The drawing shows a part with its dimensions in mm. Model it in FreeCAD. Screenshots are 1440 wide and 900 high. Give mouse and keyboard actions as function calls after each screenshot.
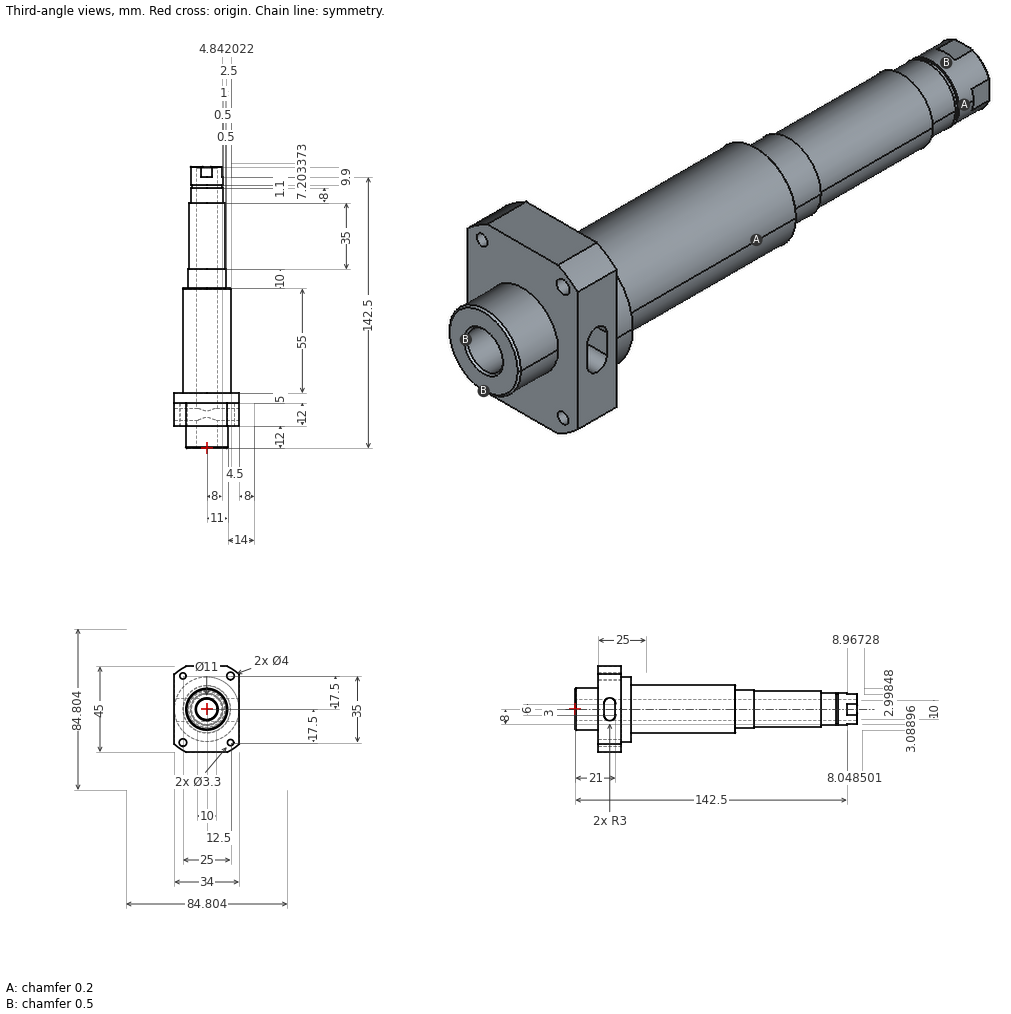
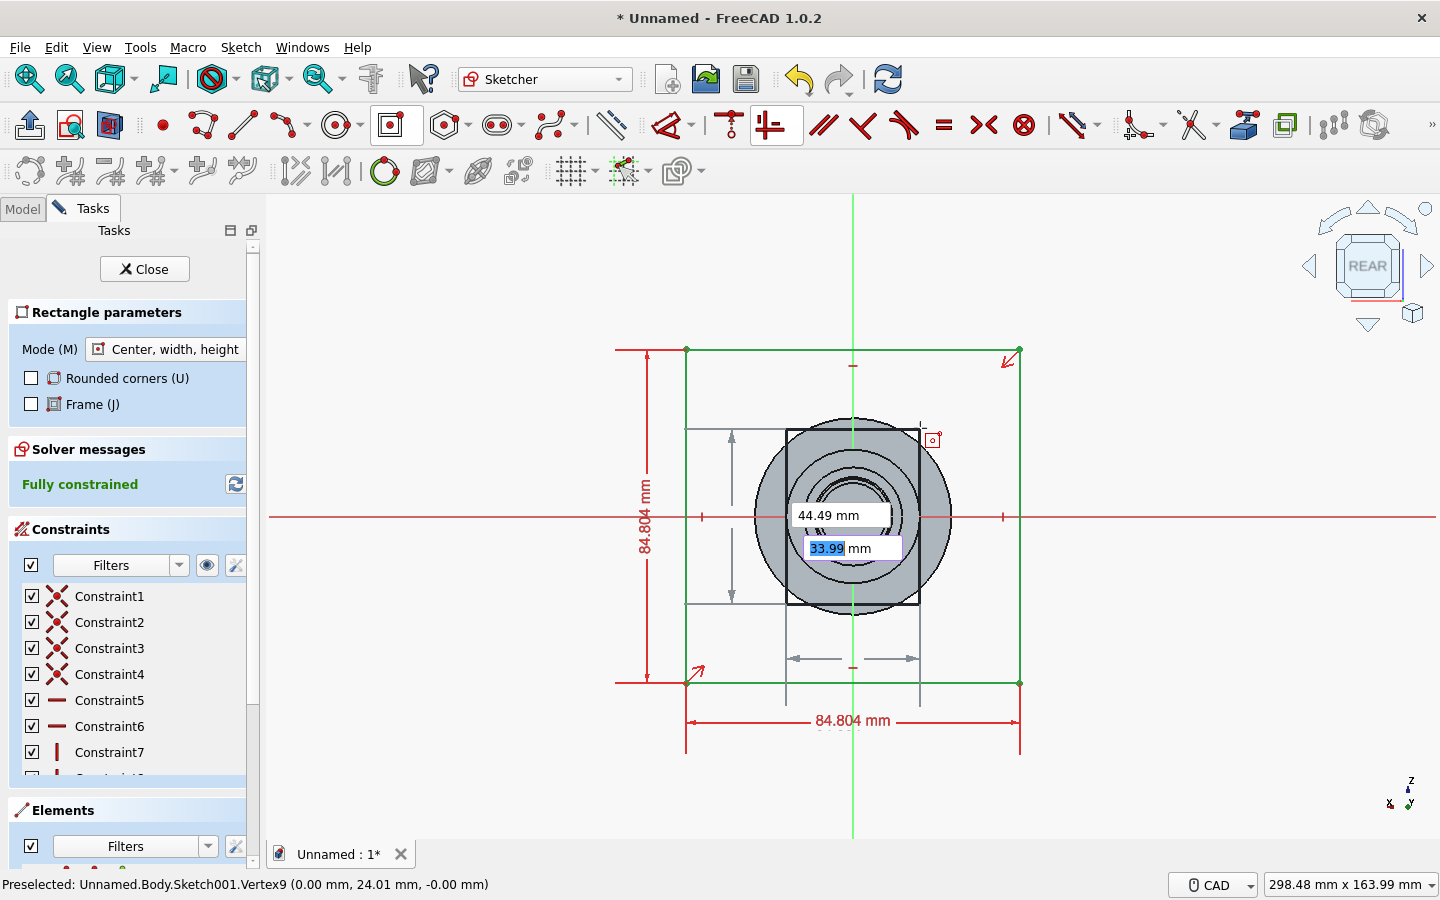
text(34)
key(Tab)
text(45)
key(Return)
key(Escape)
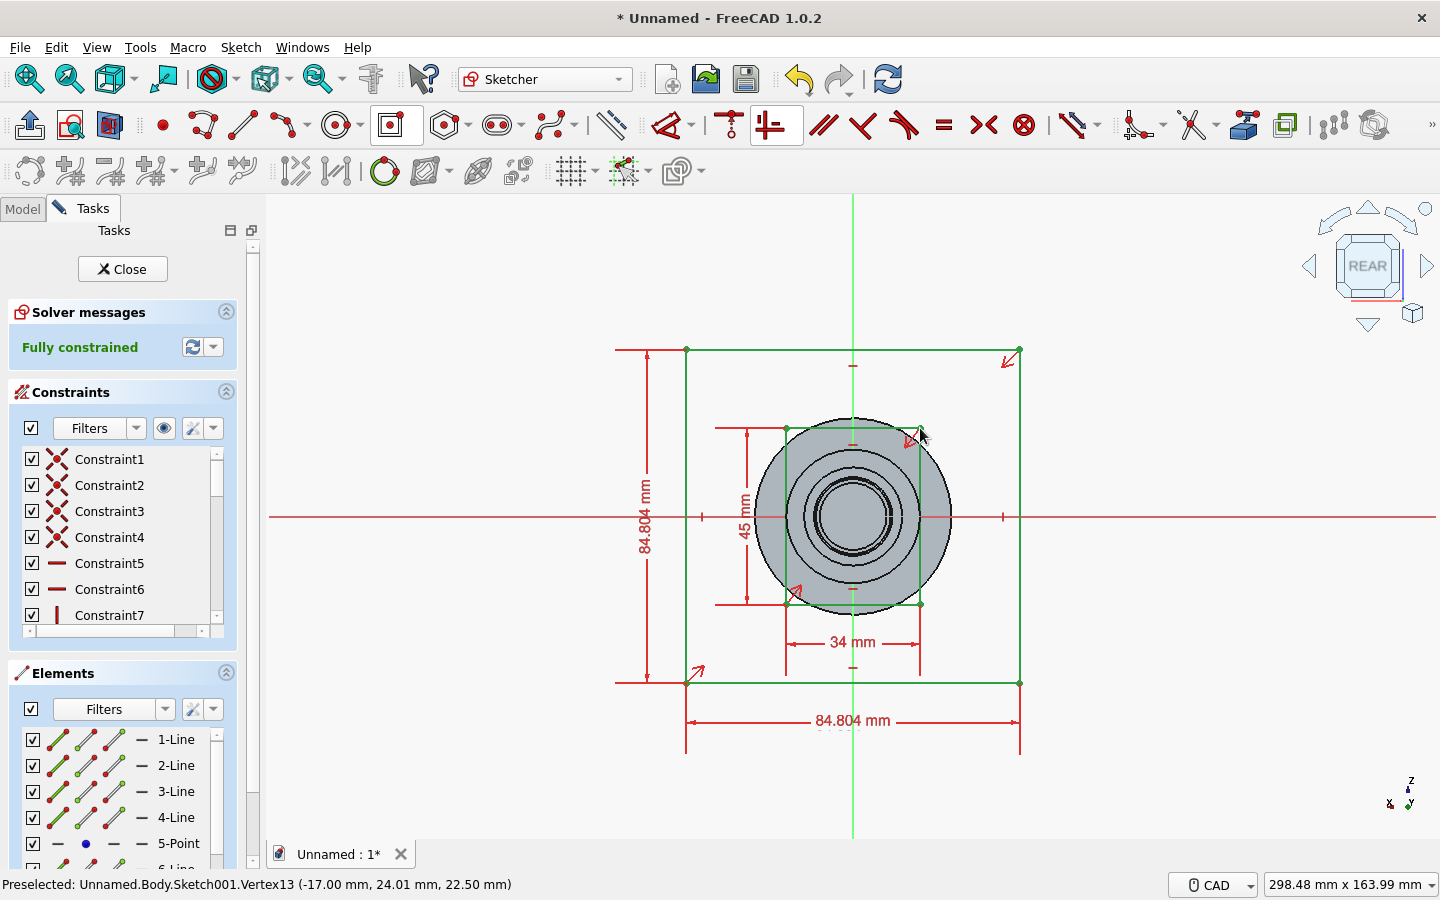
click(123, 269)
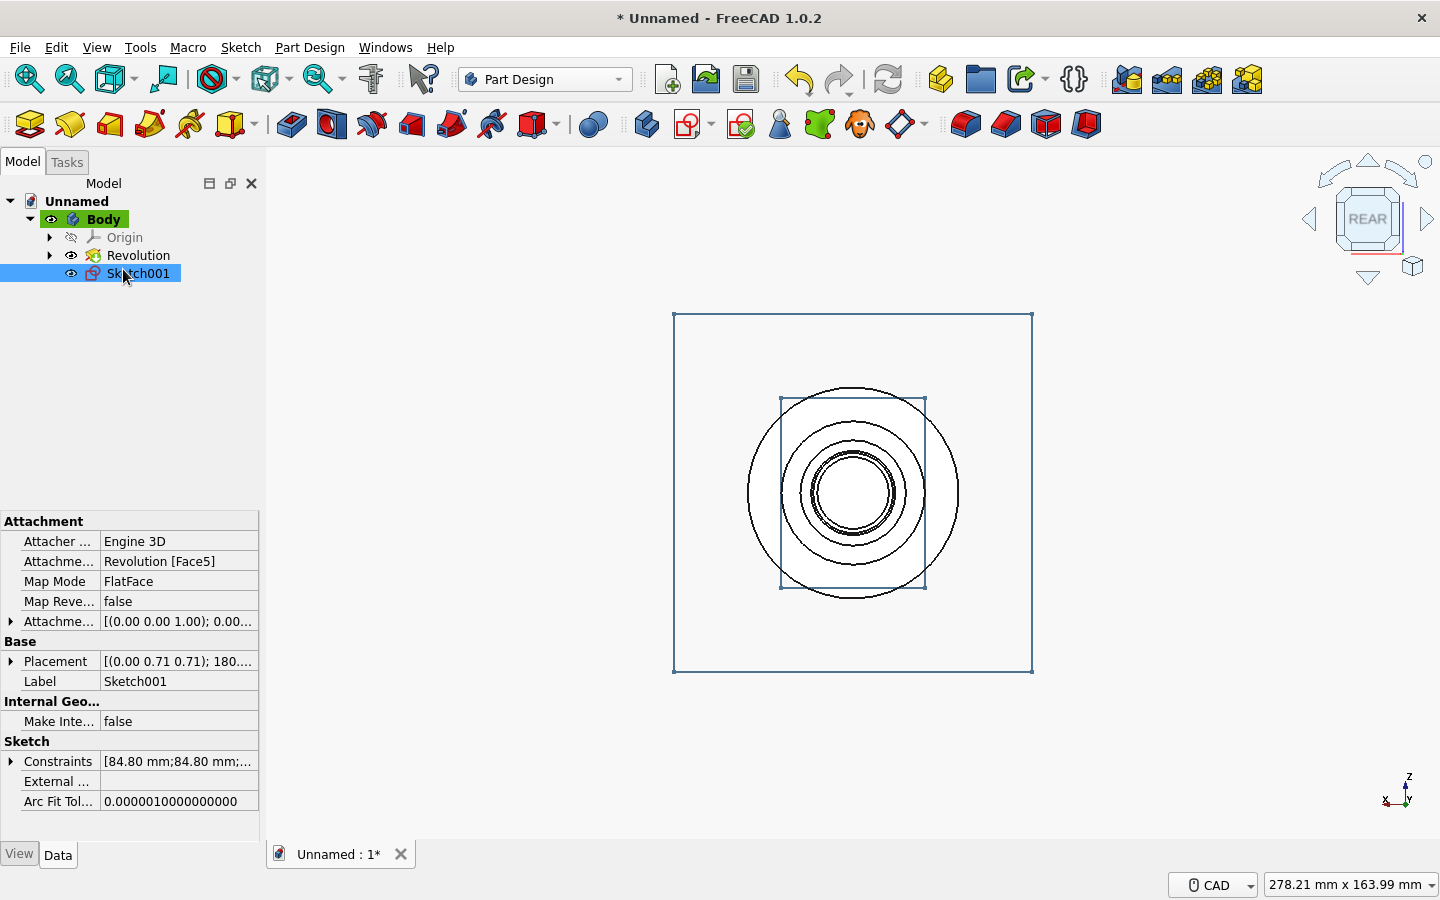
click(292, 124)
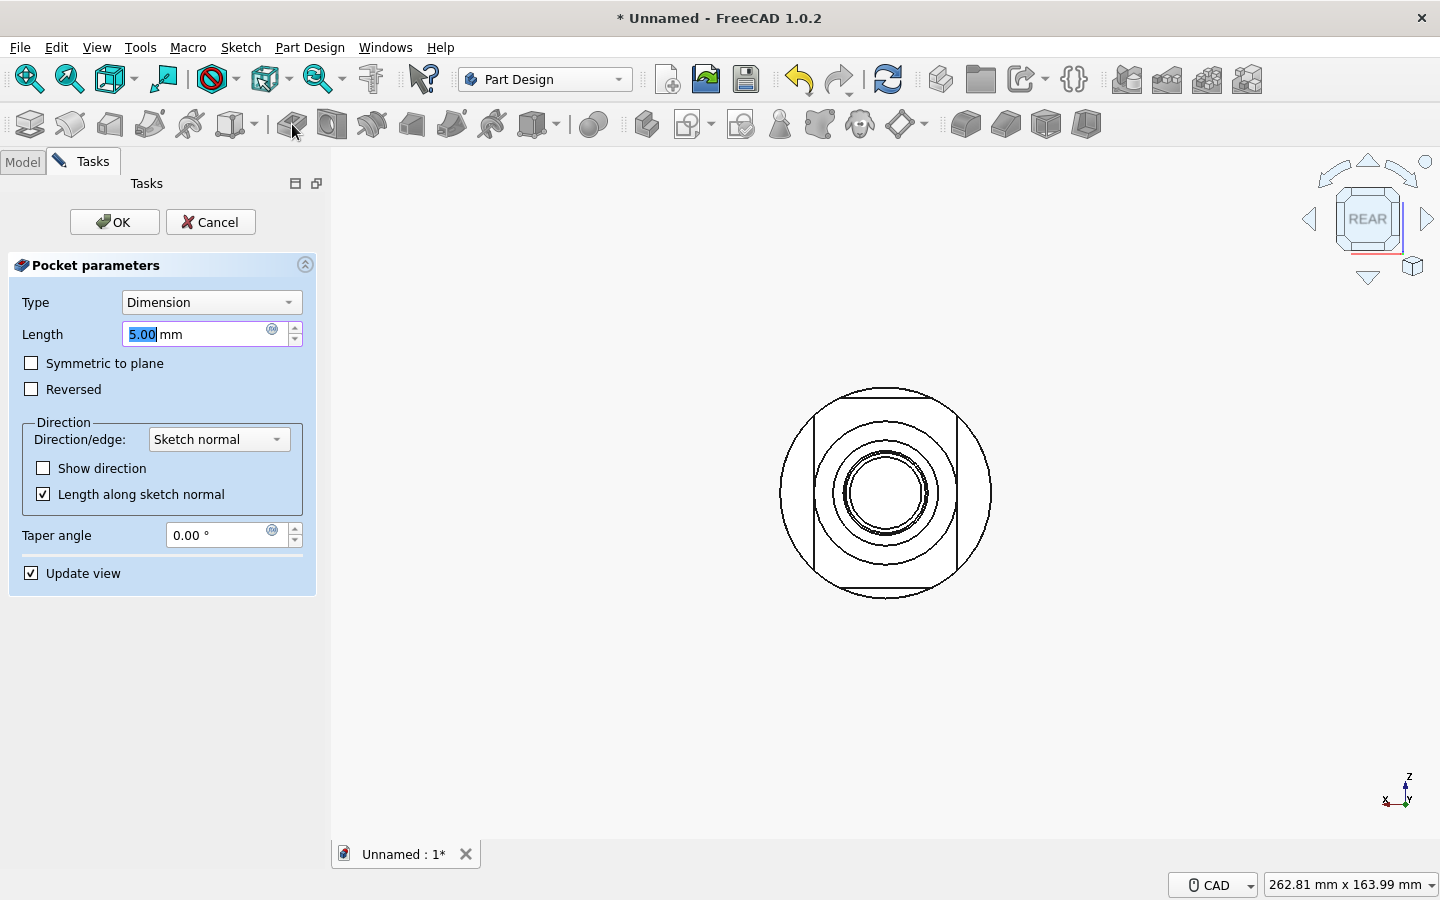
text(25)
key(Tab)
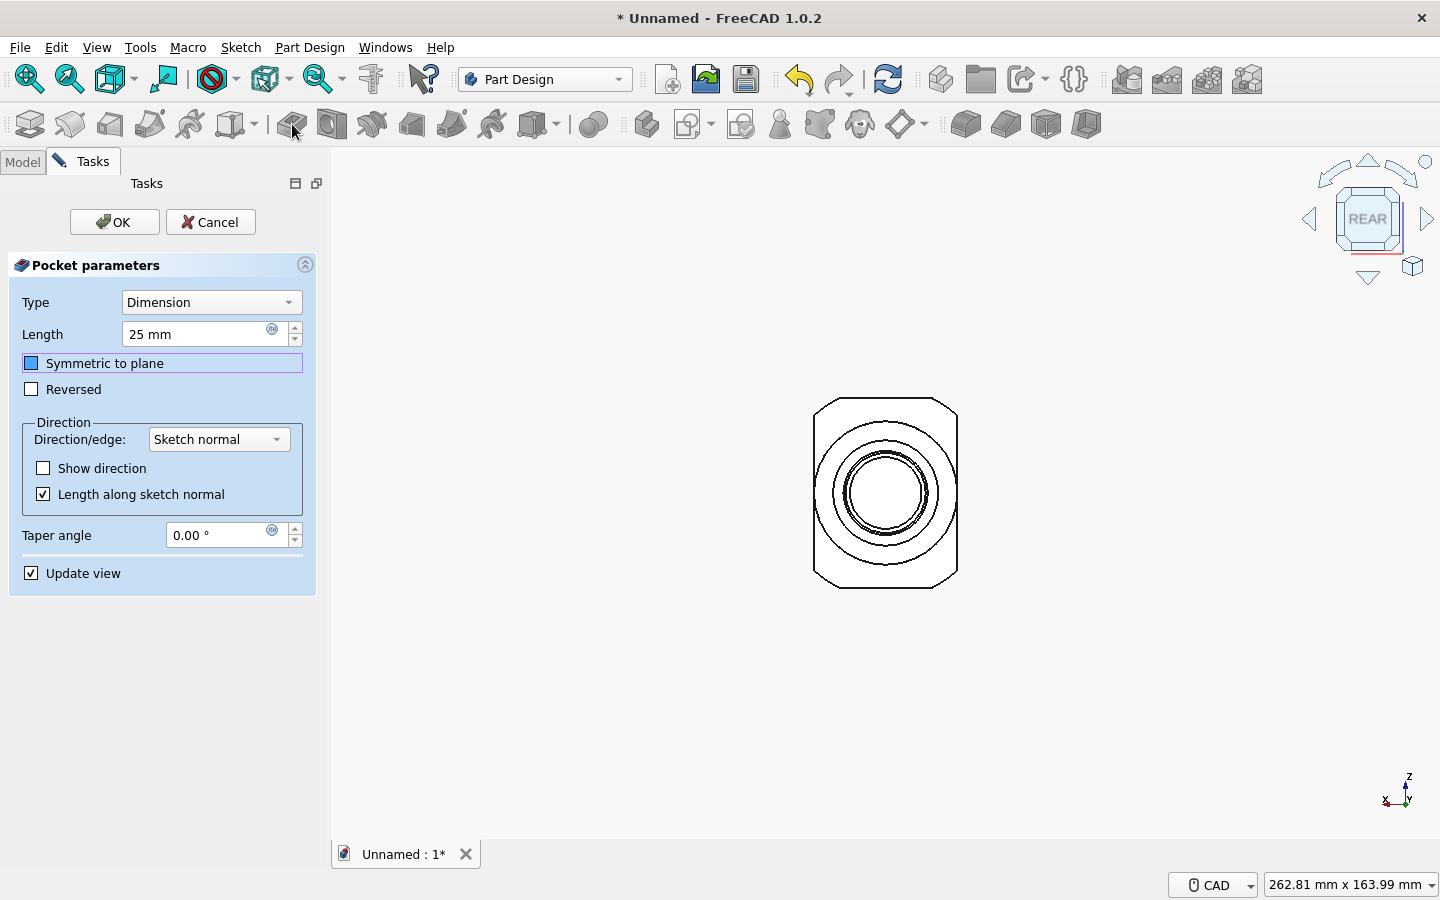
click(115, 222)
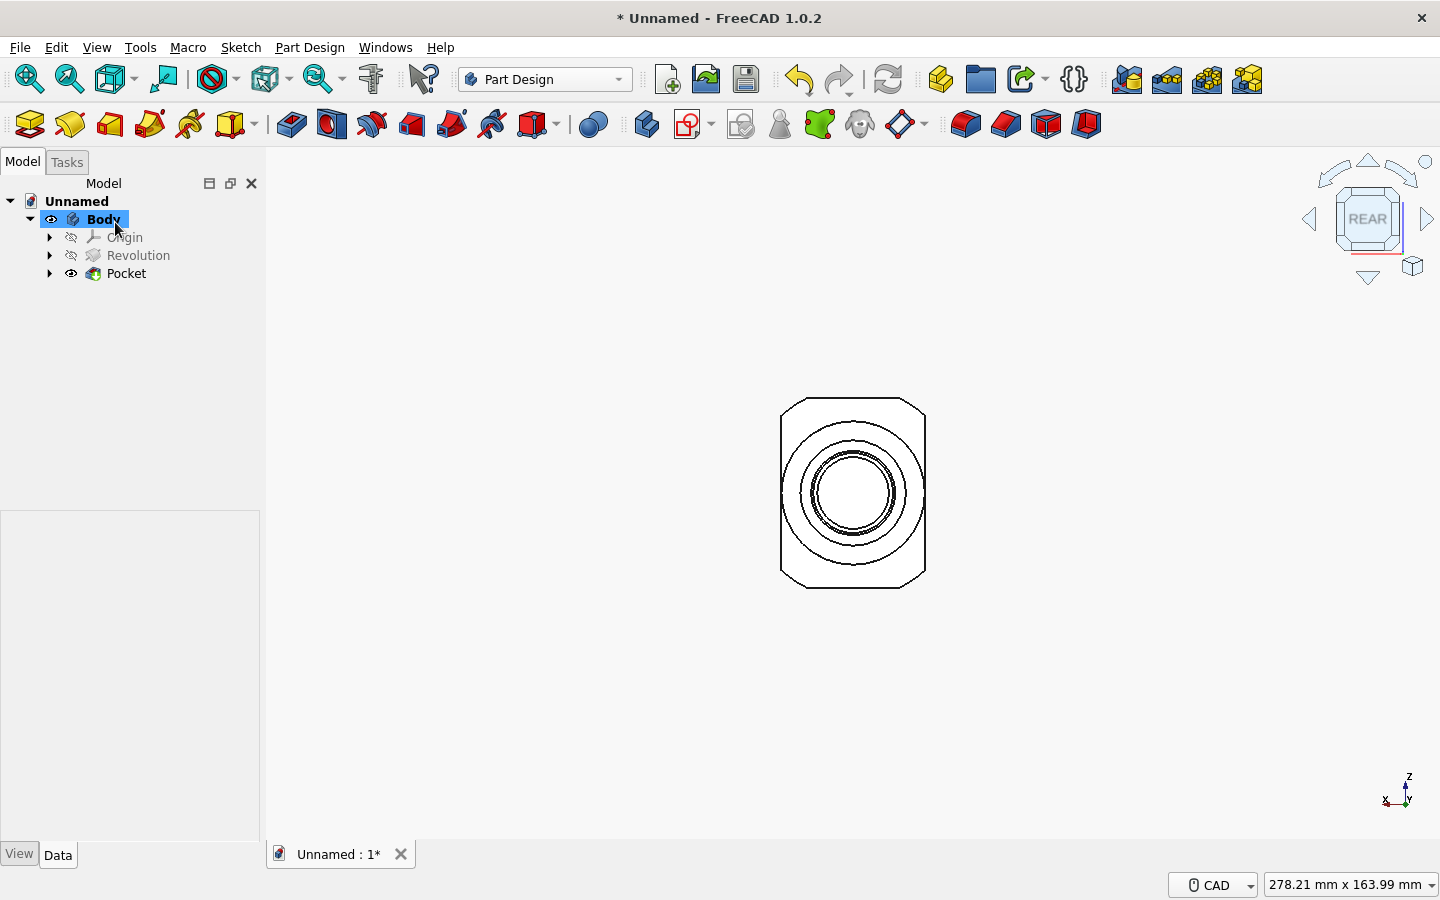
click(30, 80)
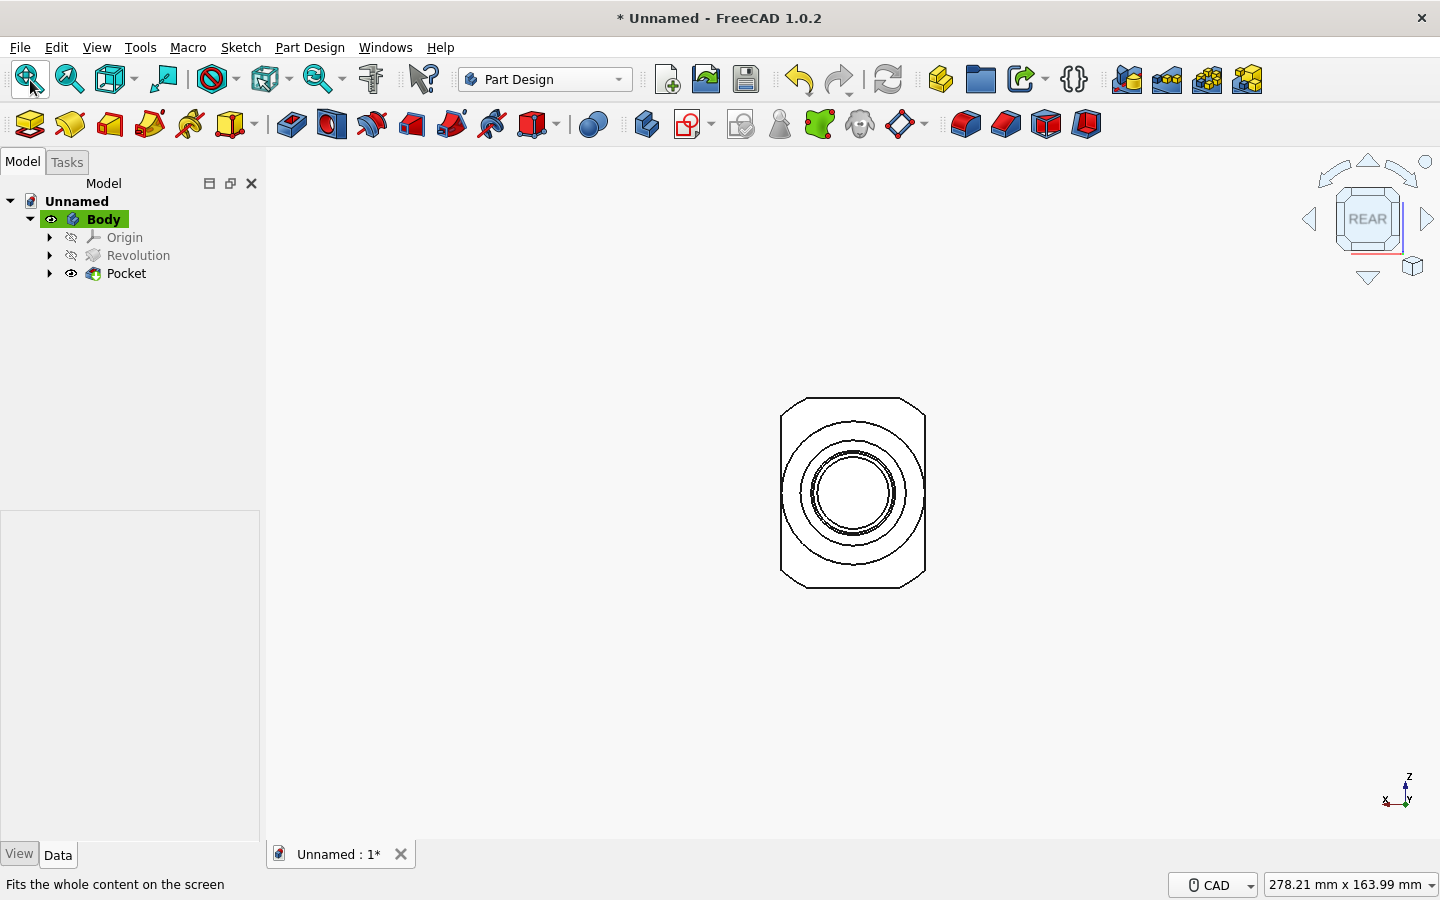
key(0)